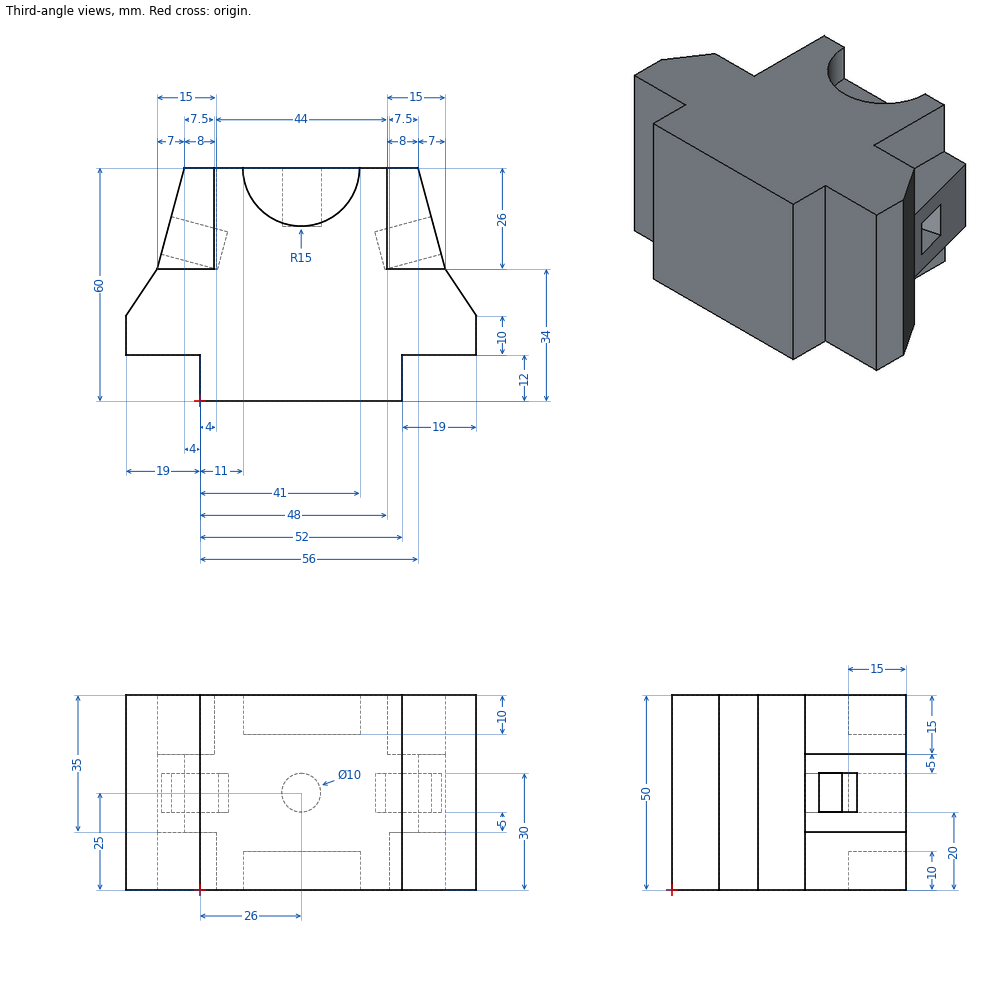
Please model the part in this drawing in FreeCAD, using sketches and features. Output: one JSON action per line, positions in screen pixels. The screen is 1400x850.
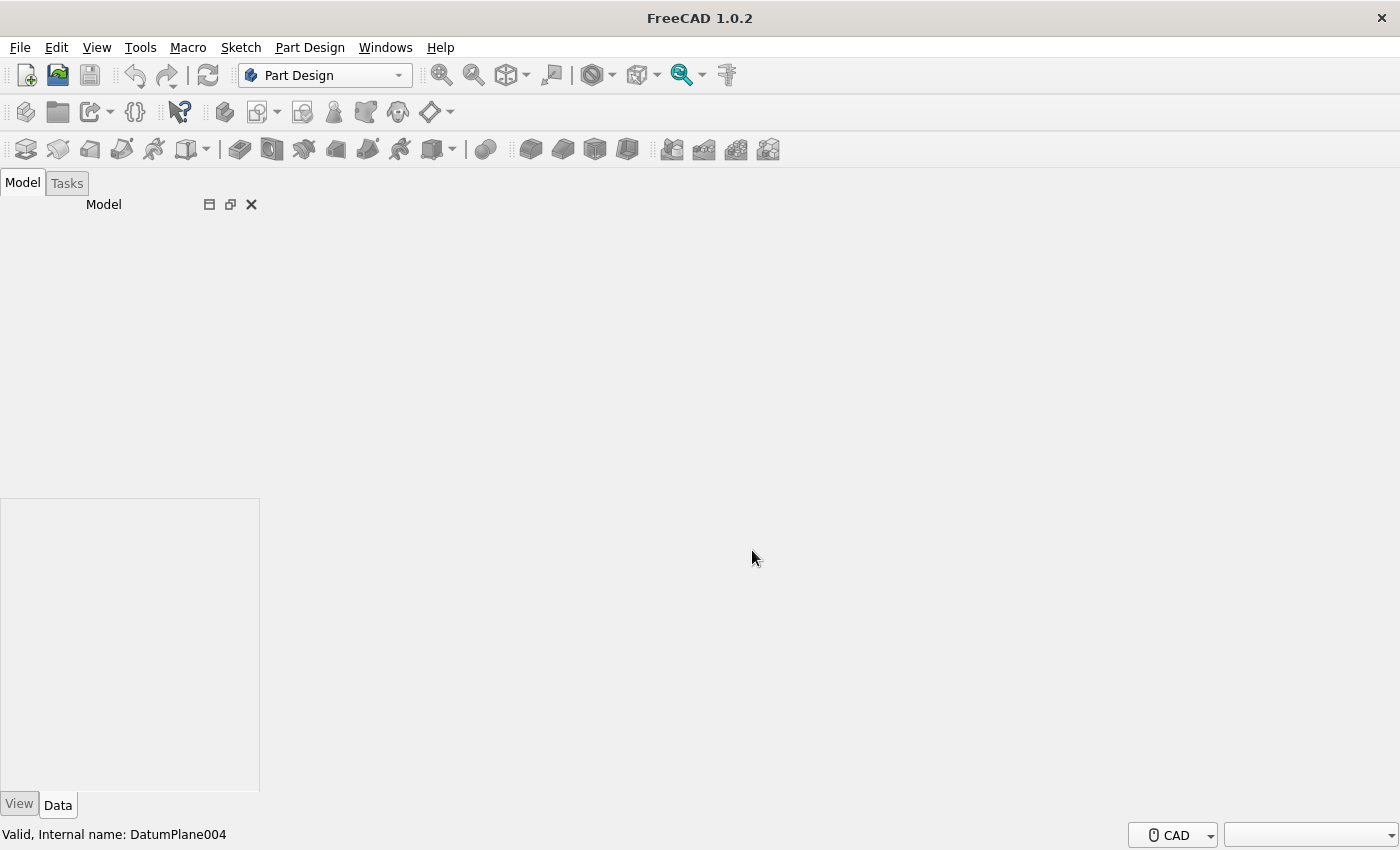
{"action": "left_click", "coordinate": [26, 76]}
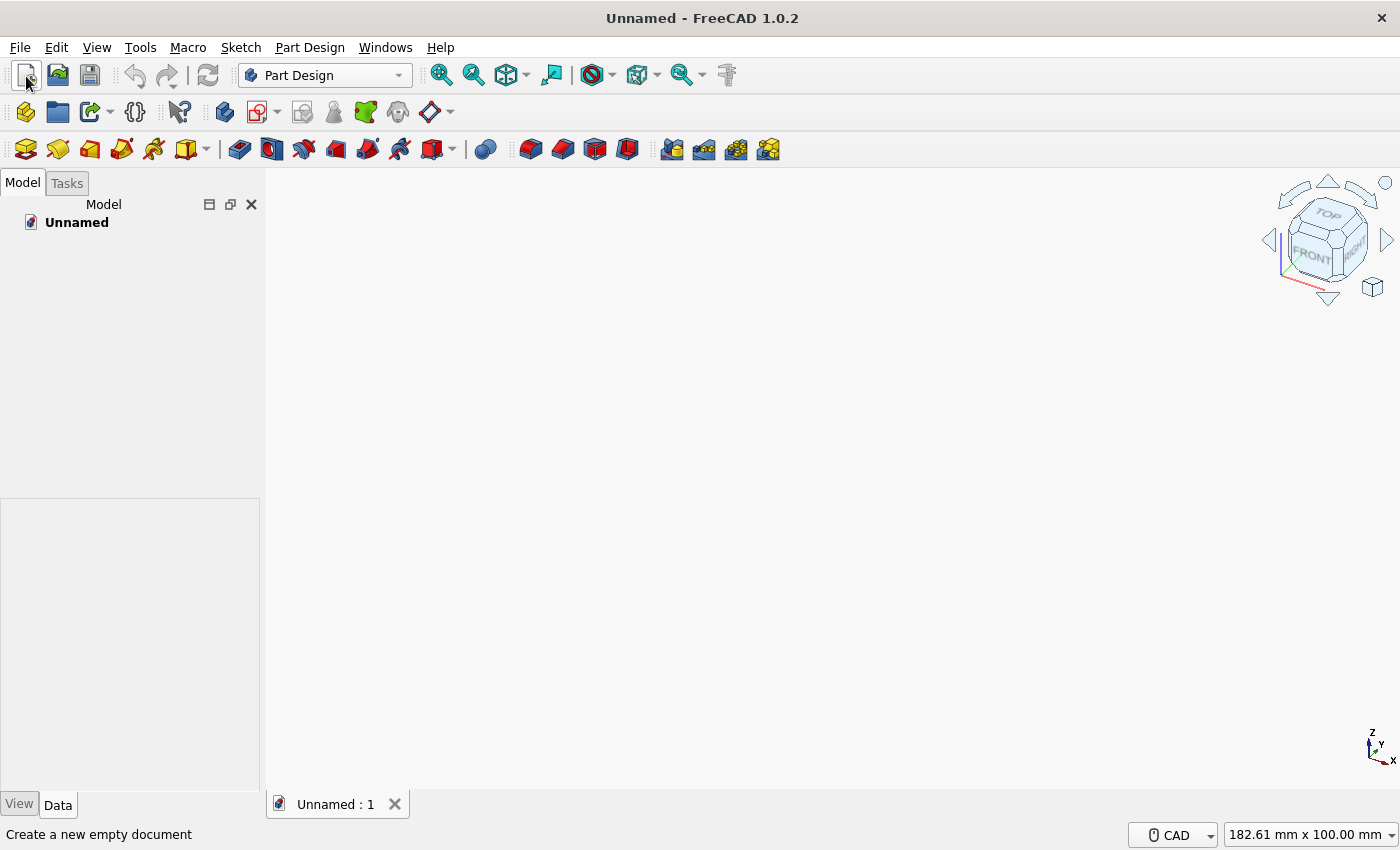
{"action": "left_click", "coordinate": [258, 112]}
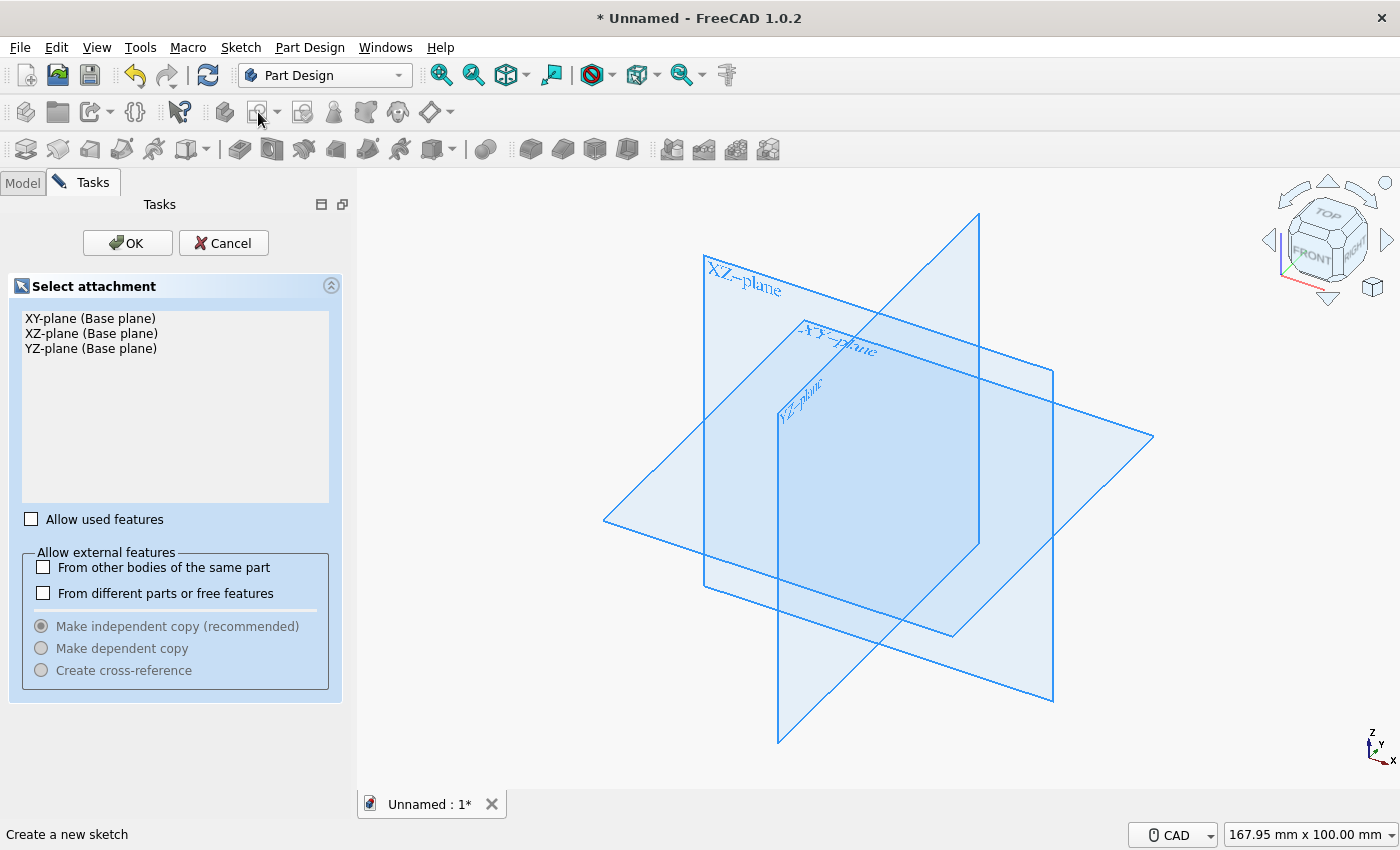
{"action": "left_click", "coordinate": [82, 318]}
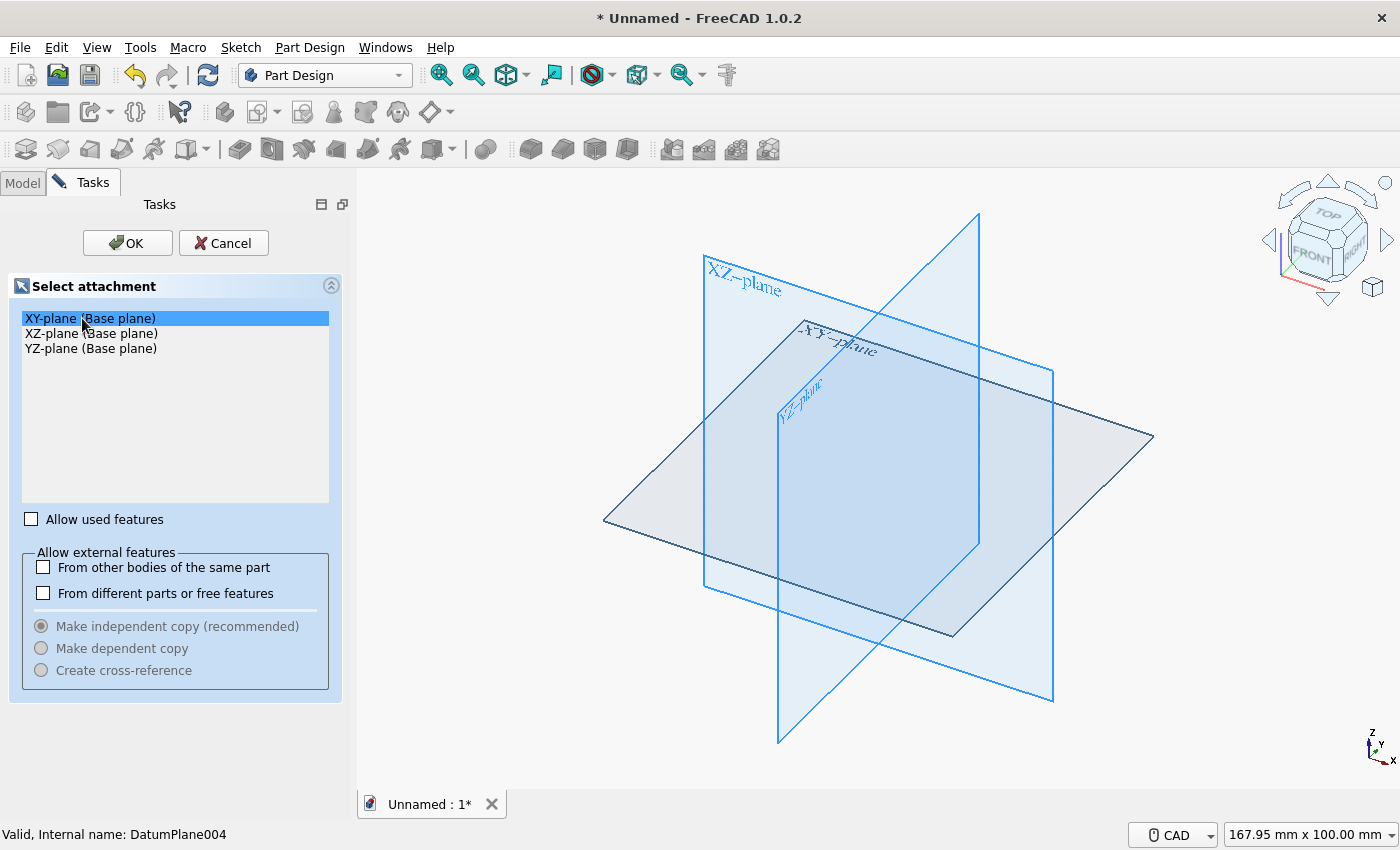
{"action": "left_click", "coordinate": [128, 243]}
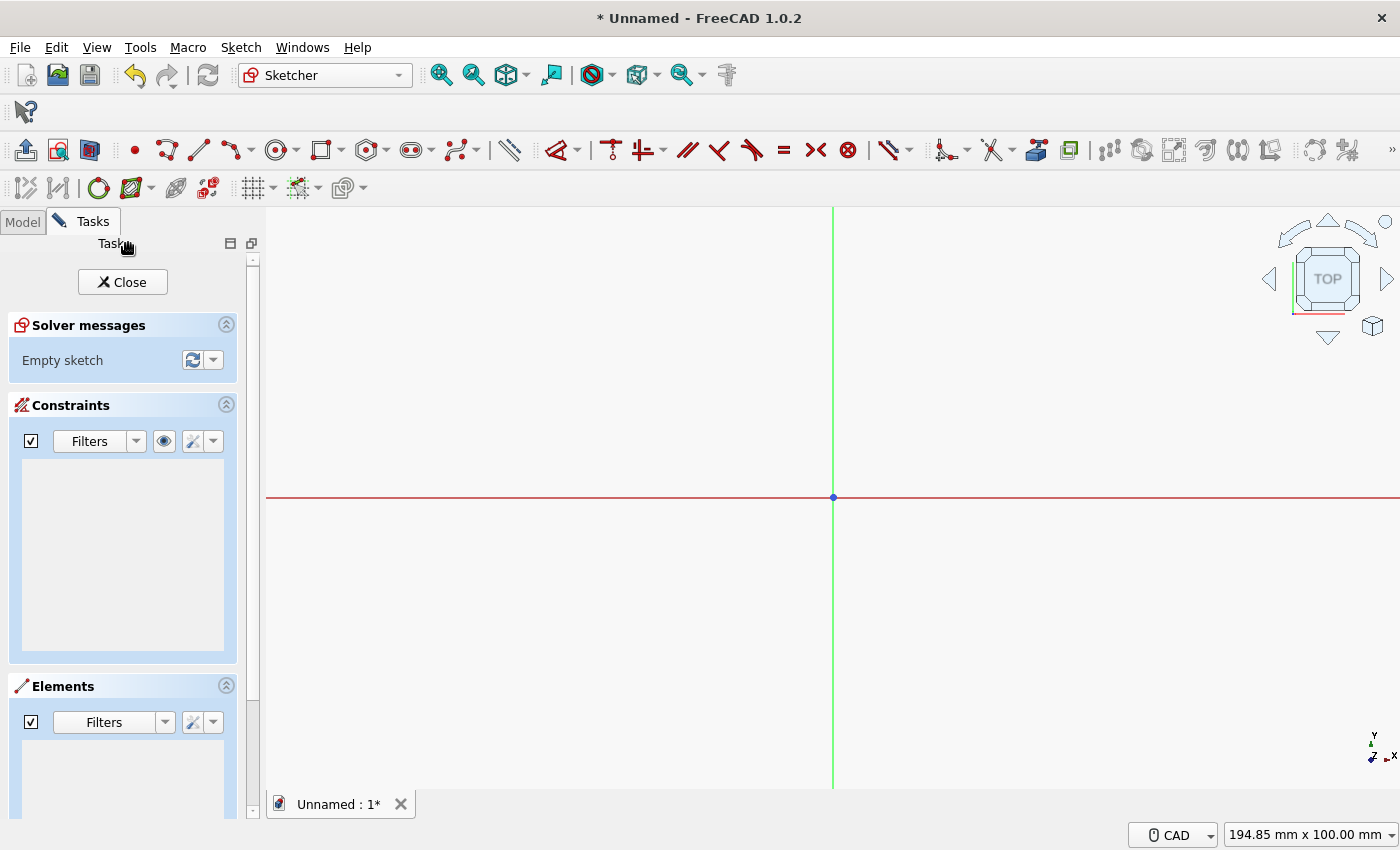
{"action": "scroll", "coordinate": [318, 761], "scroll_direction": "down", "scroll_amount": 2}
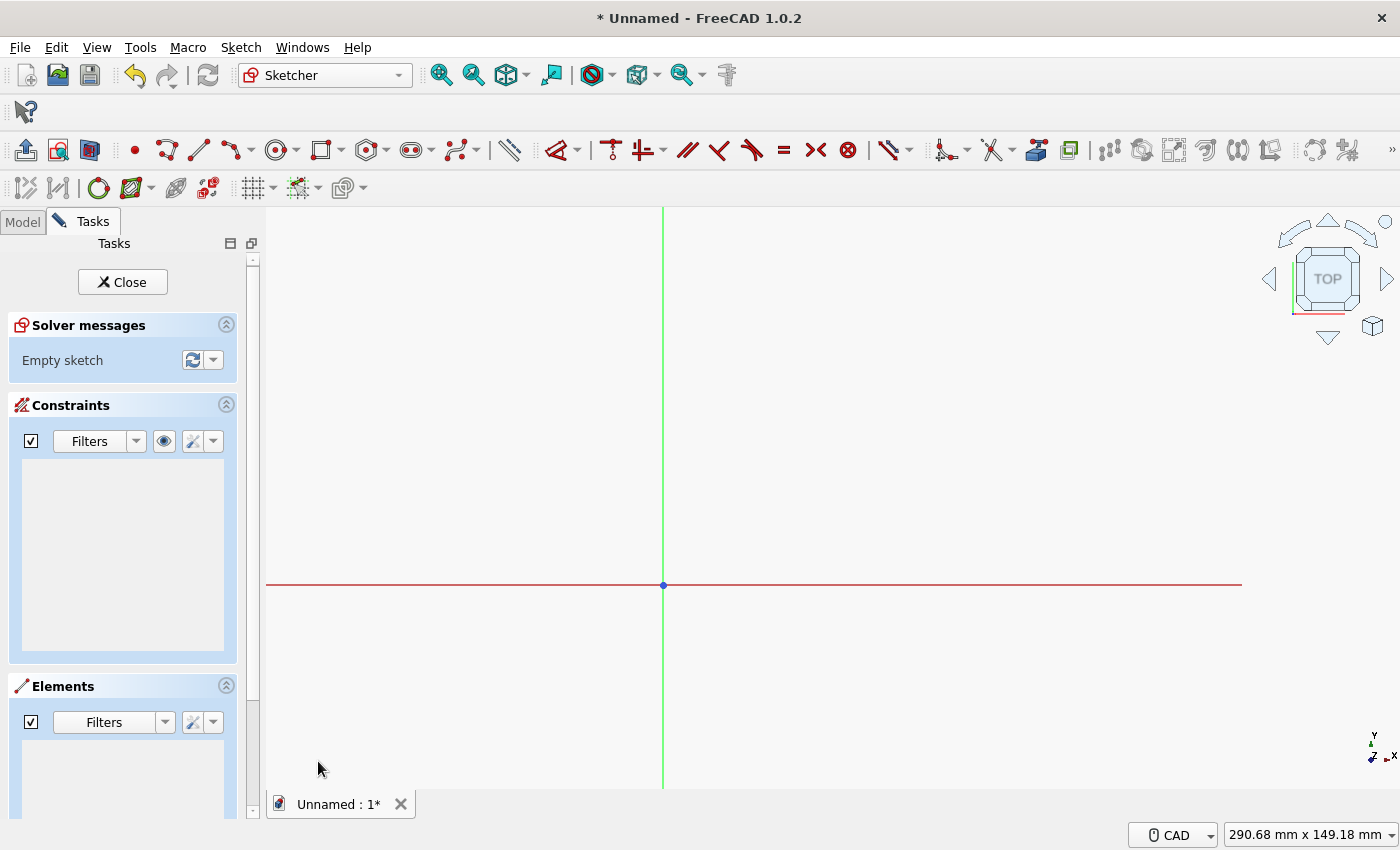
{"action": "scroll", "coordinate": [765, 407], "scroll_direction": "up", "scroll_amount": 2}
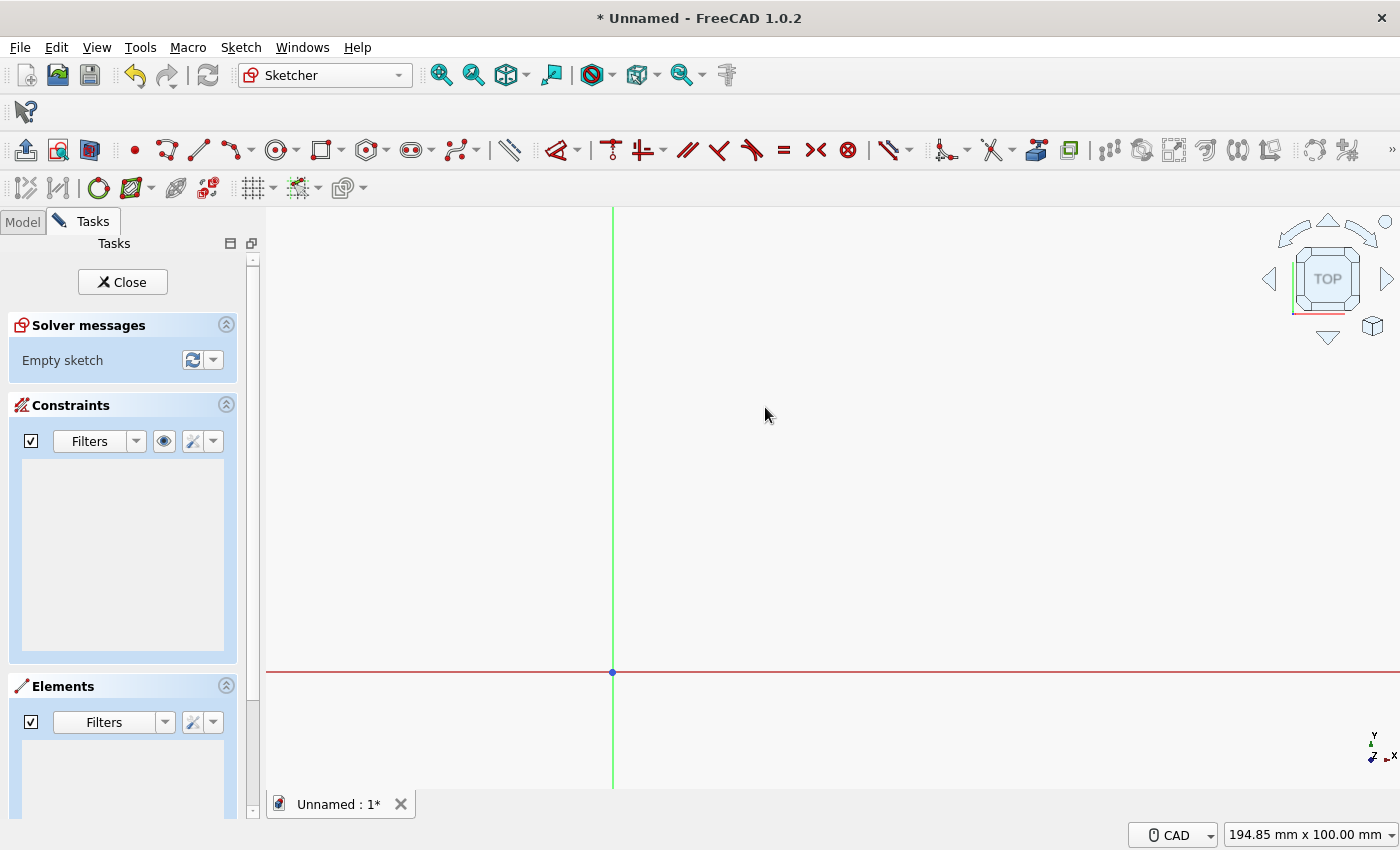
{"action": "left_click", "coordinate": [168, 150]}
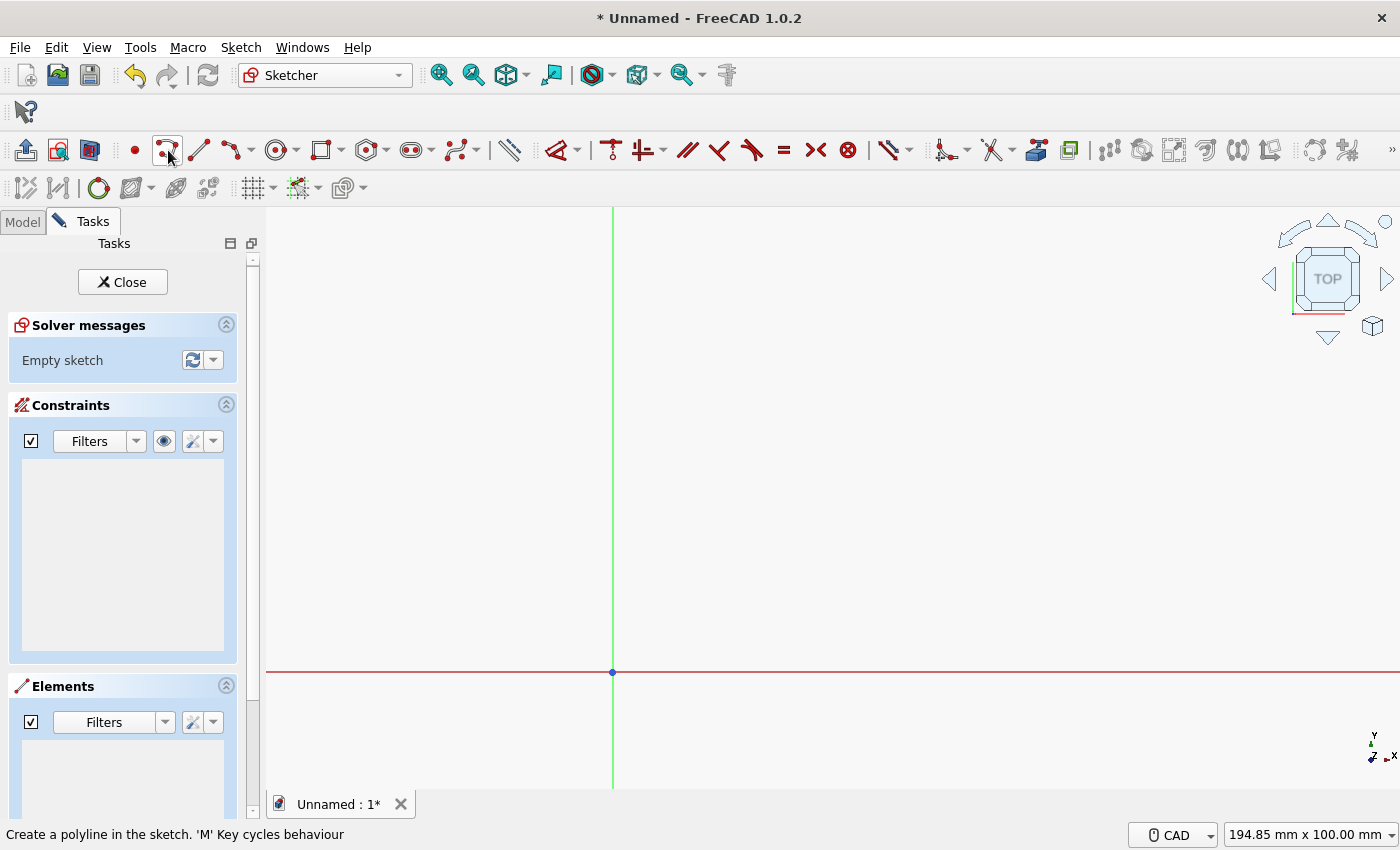
{"action": "left_click", "coordinate": [613, 672]}
{"action": "left_click", "coordinate": [916, 663]}
{"action": "left_click", "coordinate": [916, 603]}
{"action": "left_click", "coordinate": [1026, 603]}
{"action": "left_click", "coordinate": [1026, 544]}
{"action": "left_click", "coordinate": [980, 475]}
{"action": "left_click", "coordinate": [892, 475]}
{"action": "left_click", "coordinate": [892, 323]}
{"action": "left_click", "coordinate": [636, 323]}
{"action": "left_click", "coordinate": [636, 475]}
{"action": "left_click", "coordinate": [549, 475]}
{"action": "left_click", "coordinate": [502, 544]}
{"action": "left_click", "coordinate": [502, 603]}
{"action": "left_click", "coordinate": [622, 603]}
{"action": "left_click", "coordinate": [613, 672]}
{"action": "key", "text": "Escape"}
{"action": "key", "text": "Escape"}